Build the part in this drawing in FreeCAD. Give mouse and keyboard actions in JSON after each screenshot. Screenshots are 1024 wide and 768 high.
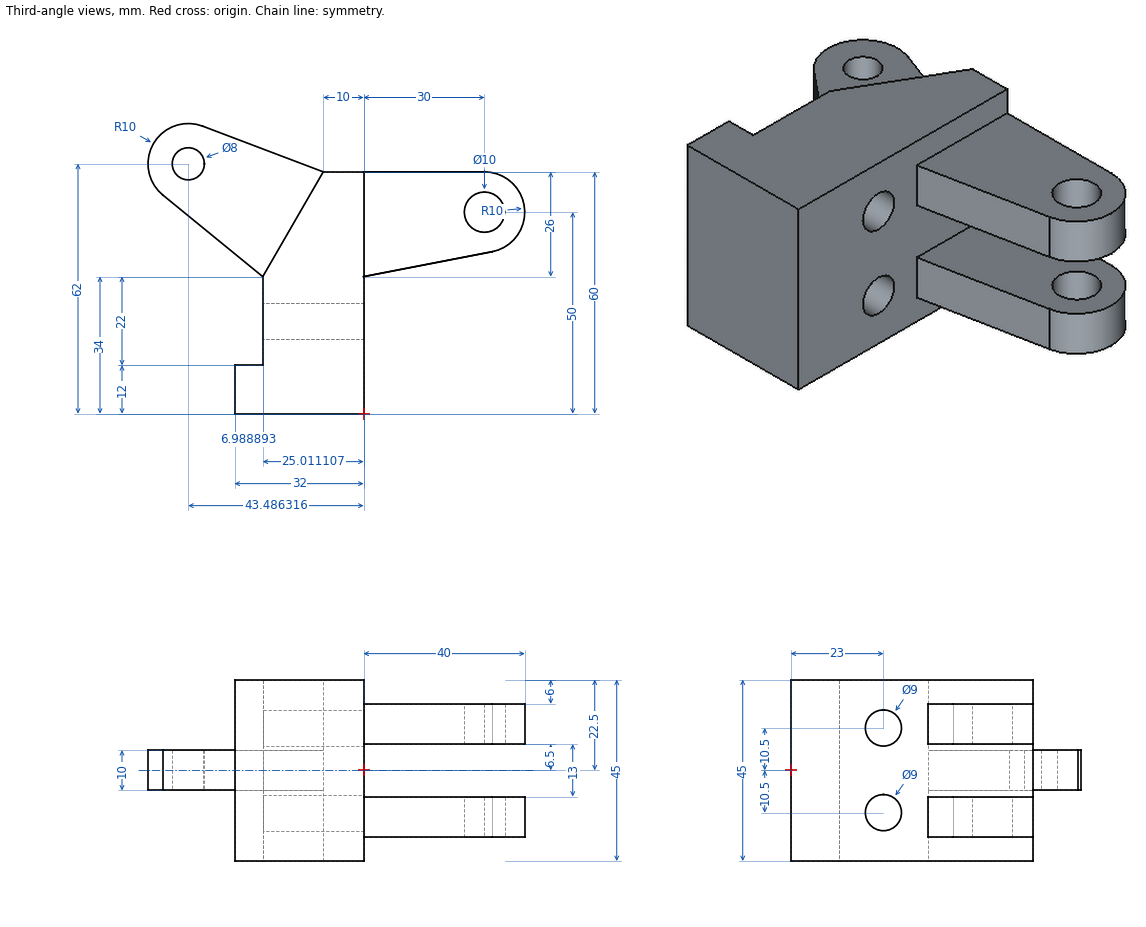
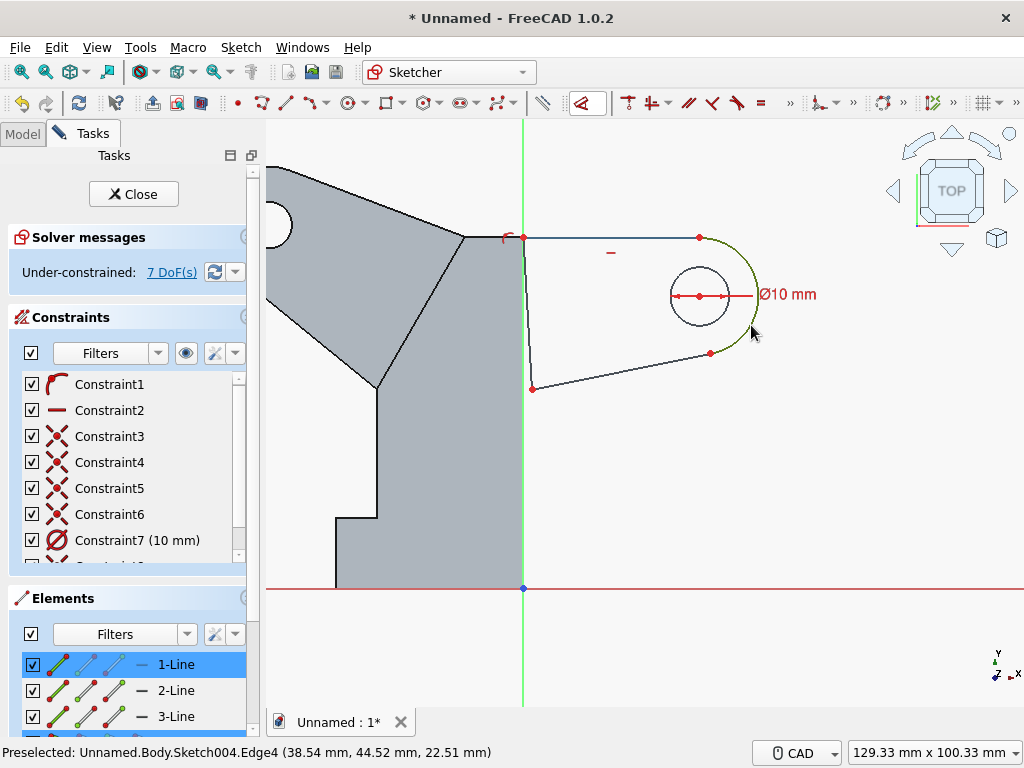
{"action": "key", "text": "t"}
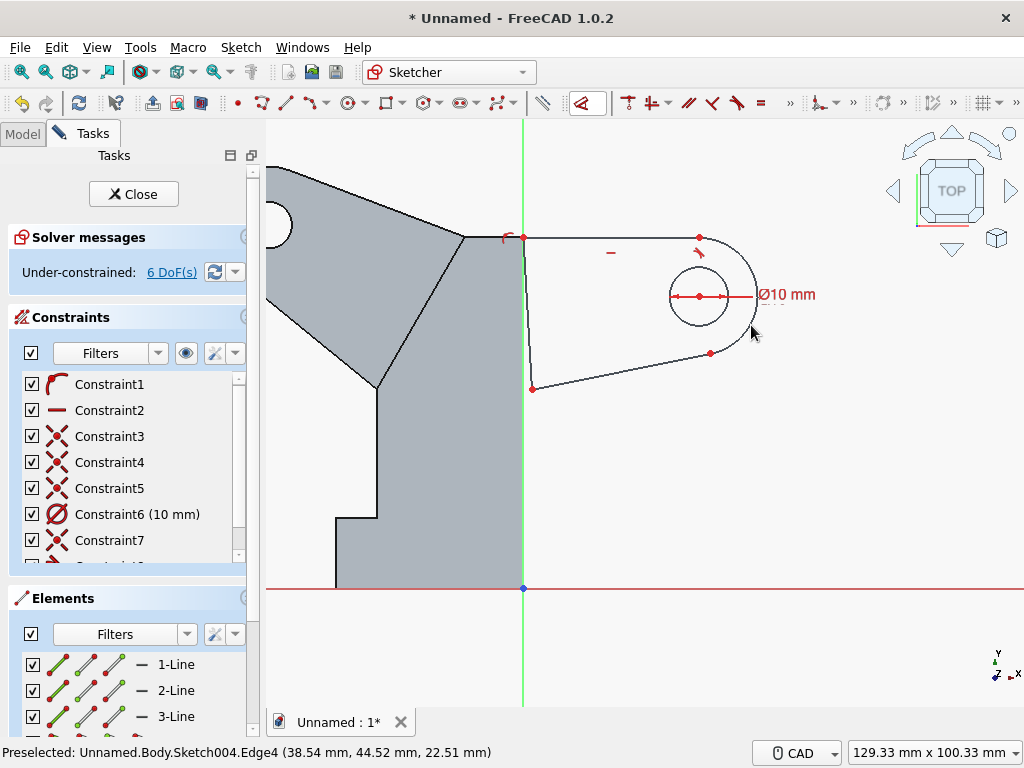
{"action": "left_click", "coordinate": [585, 379]}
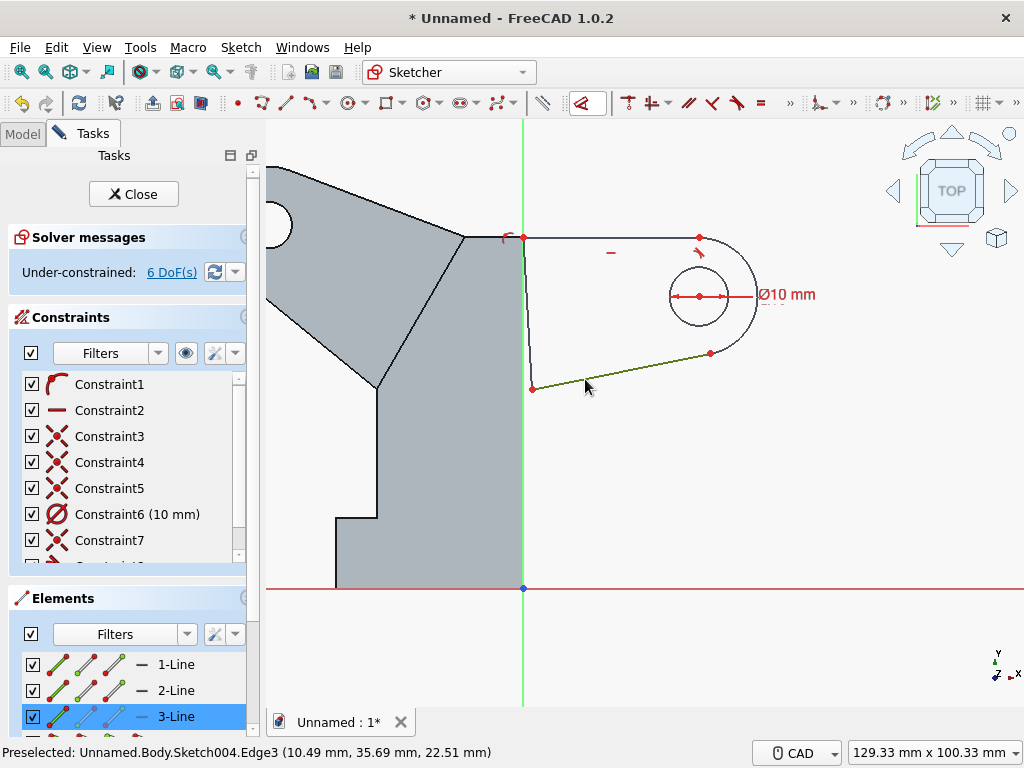
{"action": "left_click", "coordinate": [750, 324]}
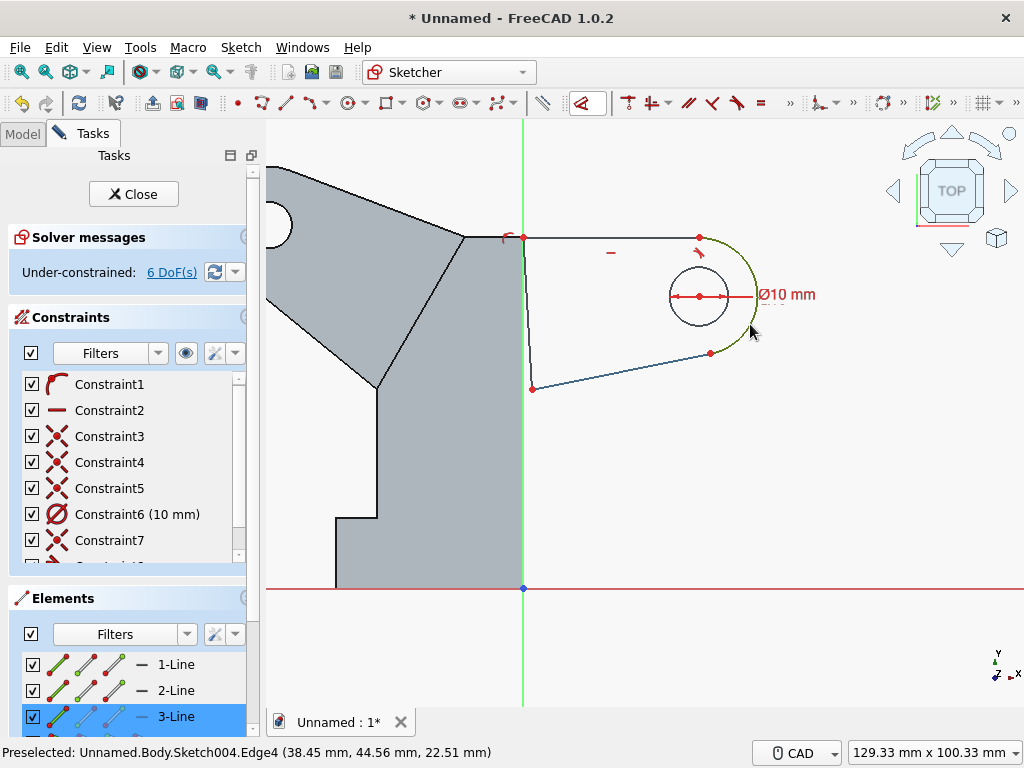
{"action": "key", "text": "t"}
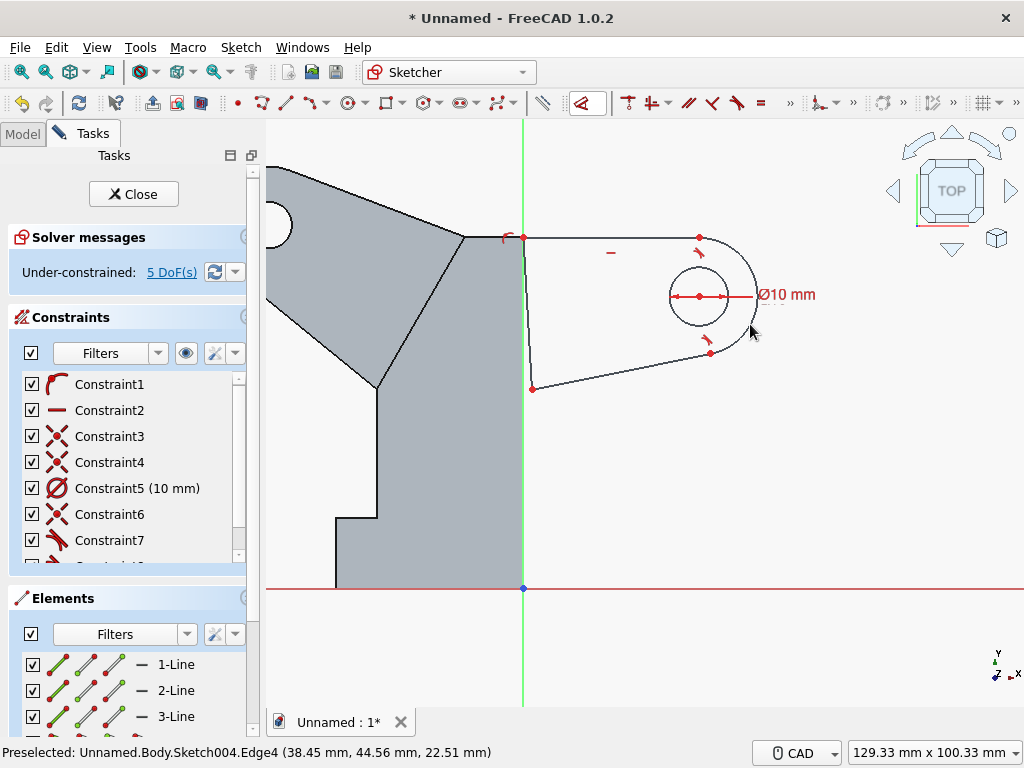
{"action": "left_click", "coordinate": [526, 284]}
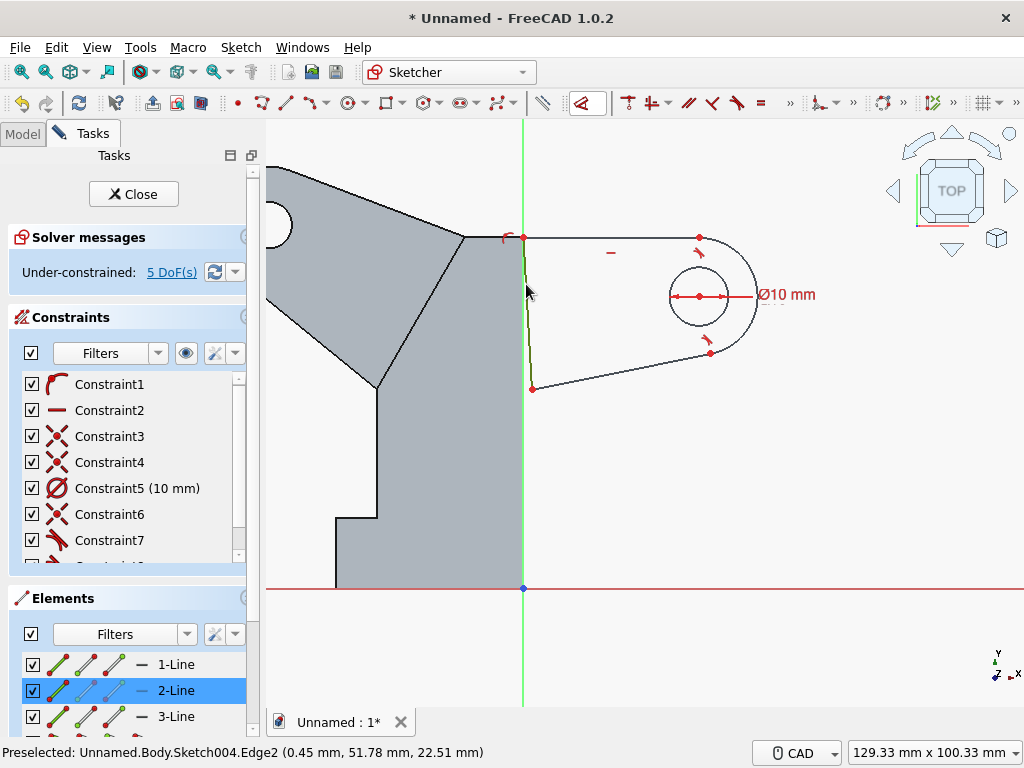
{"action": "key", "text": "v"}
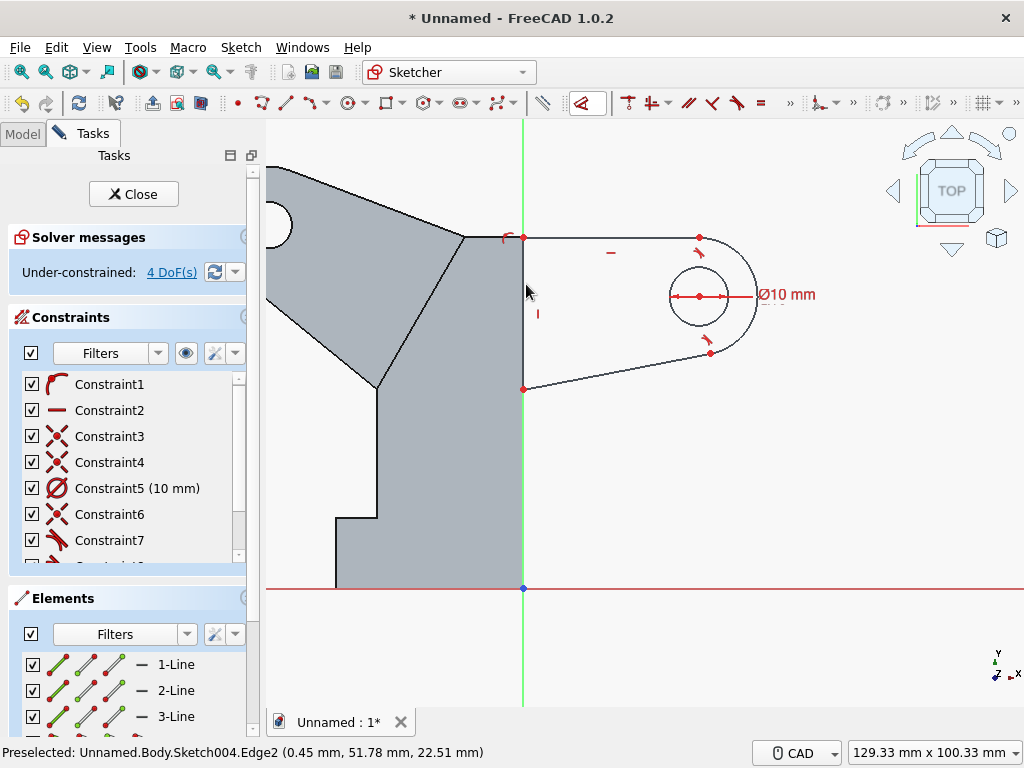
{"action": "left_click", "coordinate": [751, 324]}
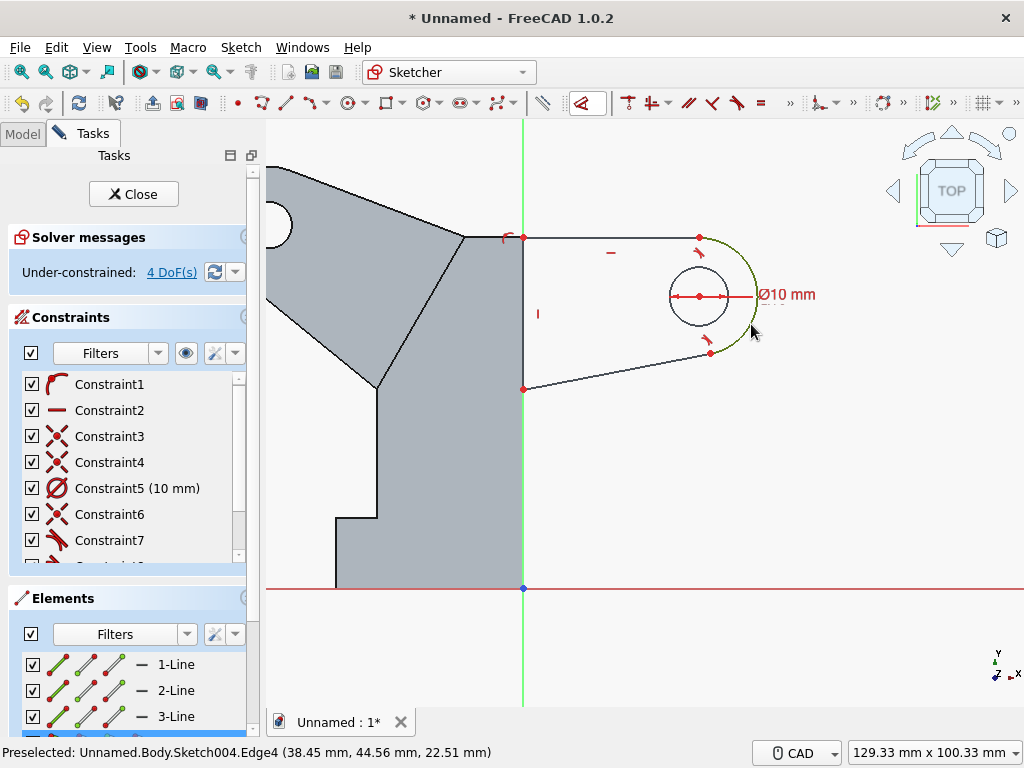
{"action": "key", "text": "k r"}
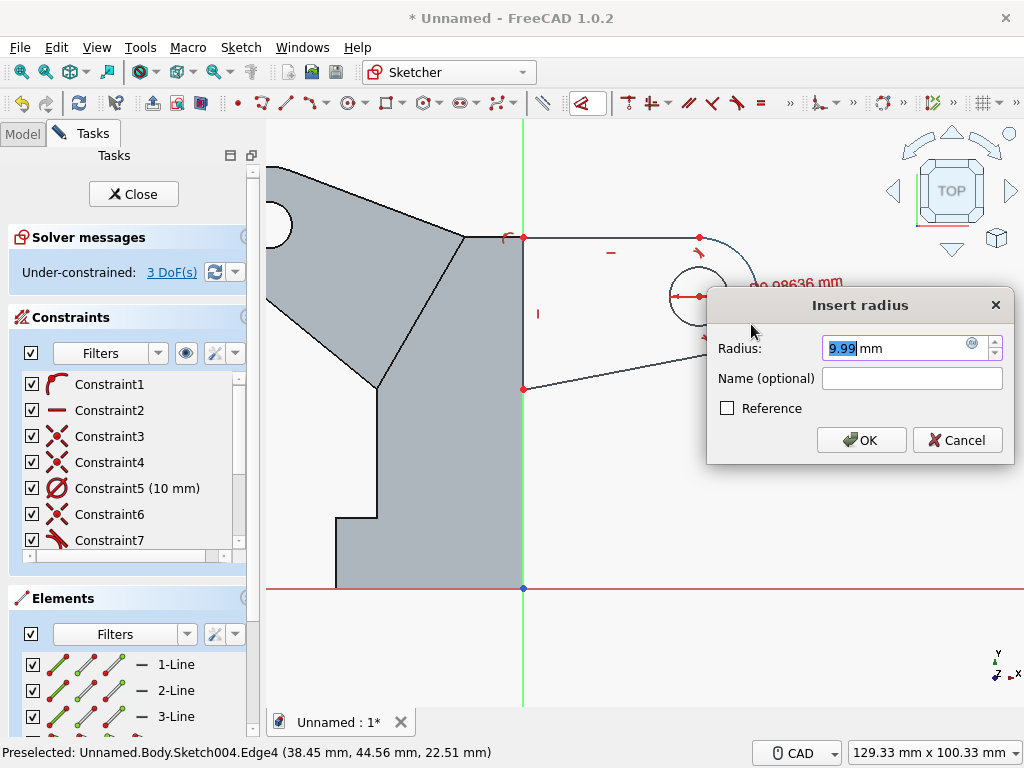
{"action": "type", "text": "10"}
{"action": "key", "text": "Return"}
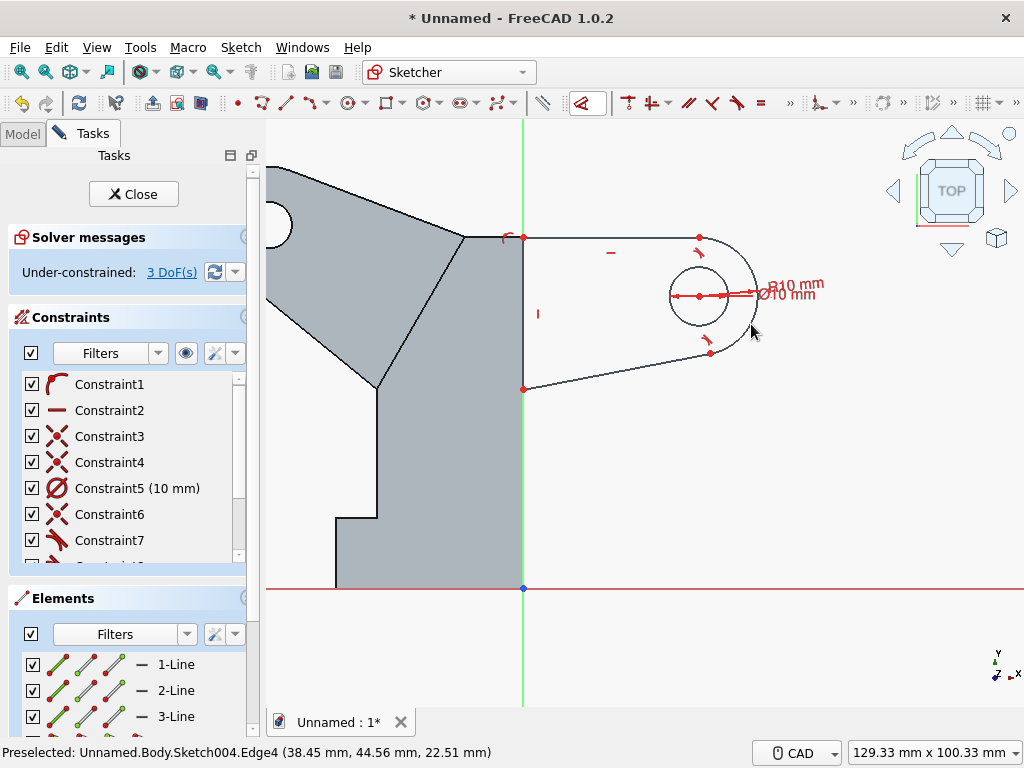
{"action": "left_click", "coordinate": [646, 238]}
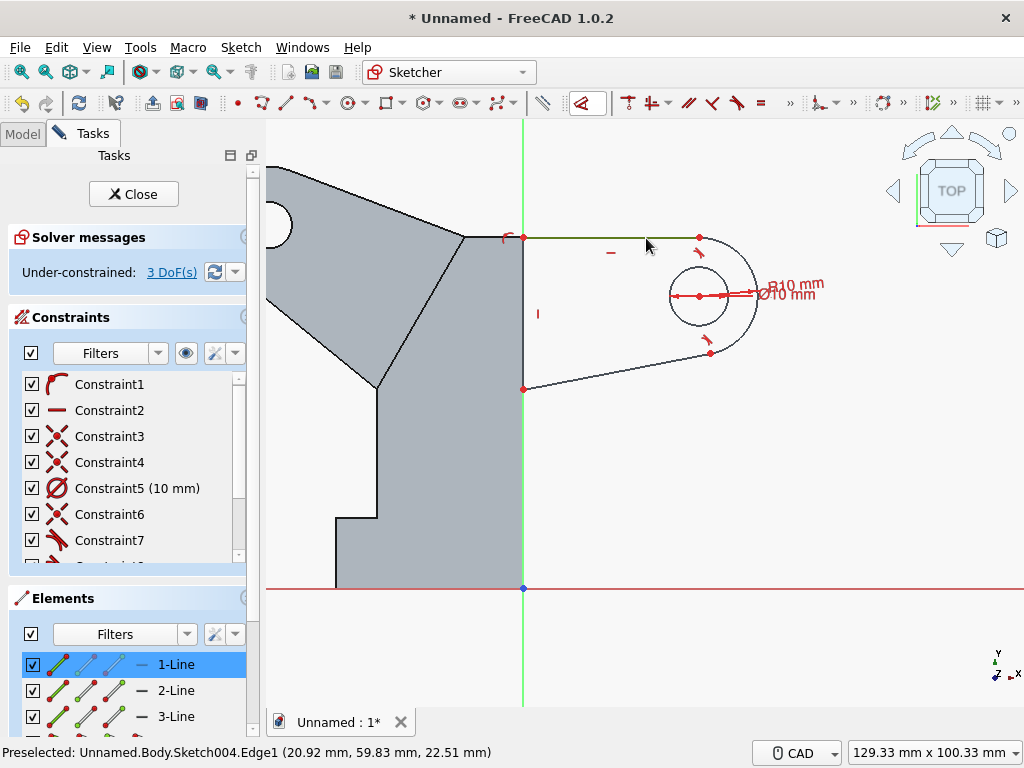
{"action": "key", "text": "l"}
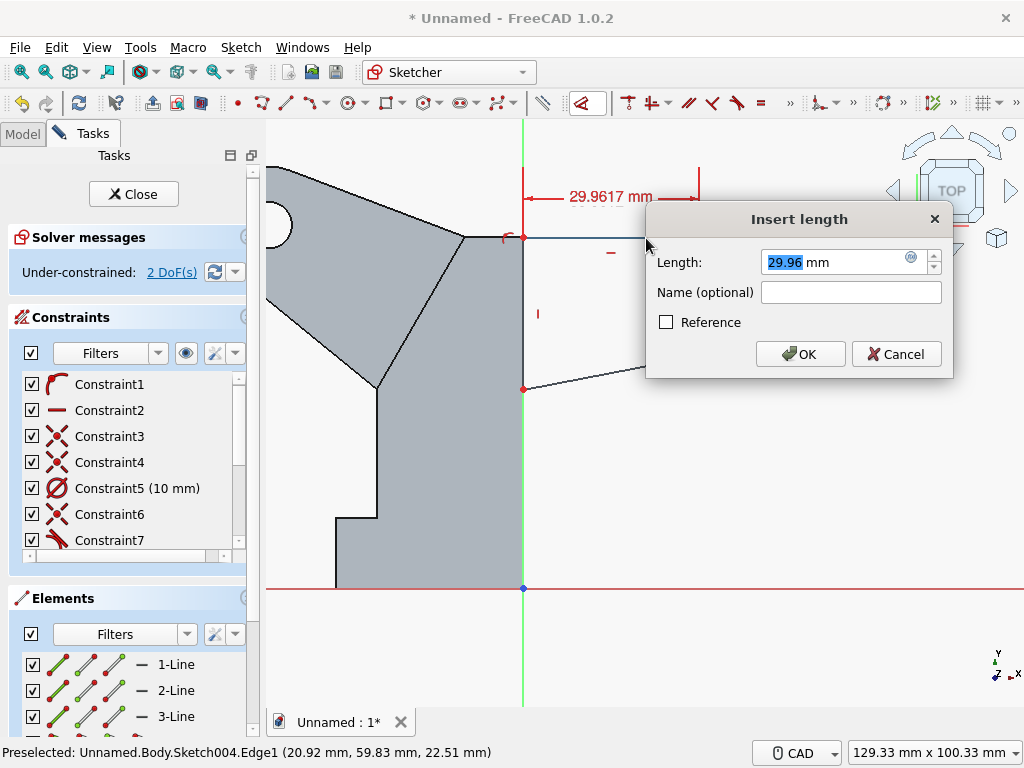
{"action": "type", "text": "30"}
{"action": "key", "text": "Return"}